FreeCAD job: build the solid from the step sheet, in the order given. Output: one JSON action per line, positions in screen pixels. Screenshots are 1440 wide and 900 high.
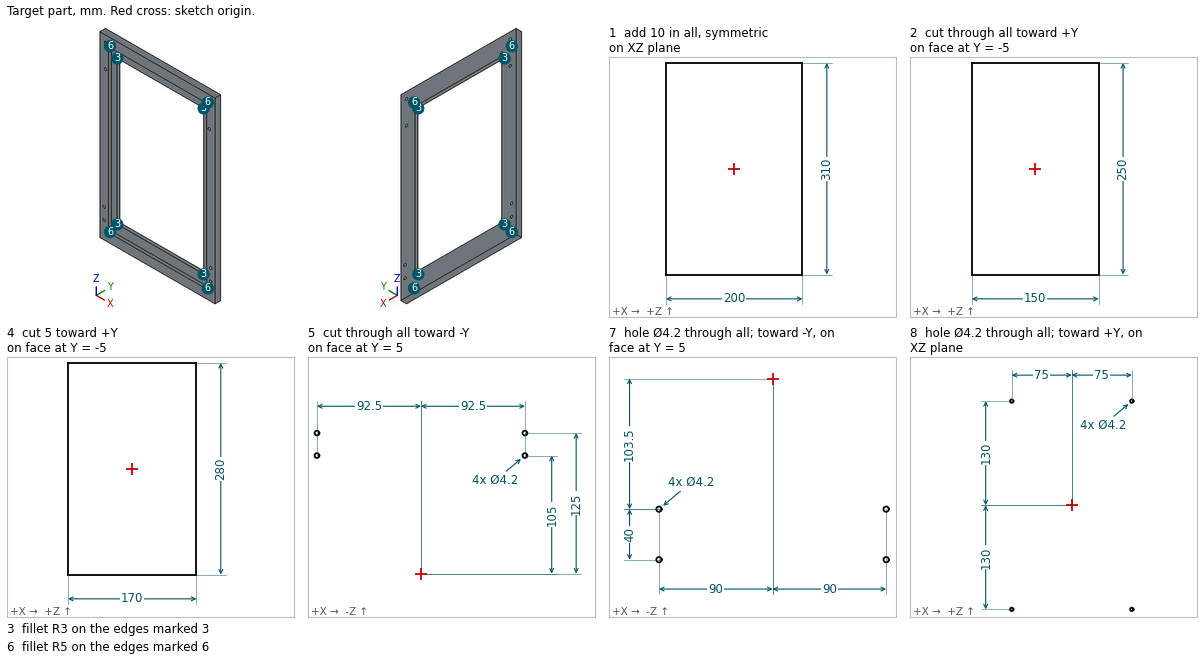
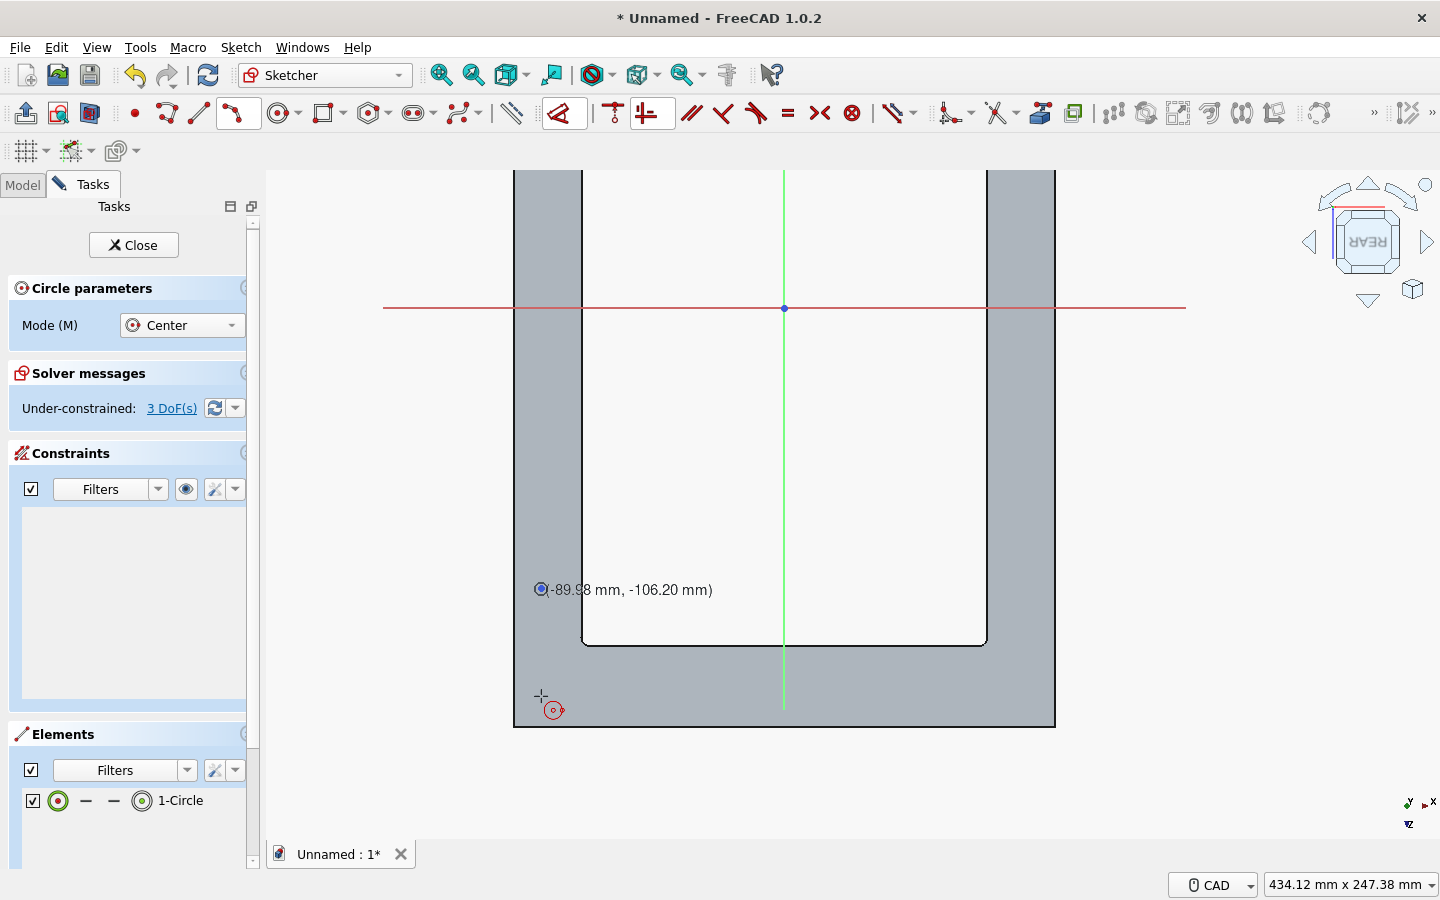
{"action": "left_click", "coordinate": [541, 696]}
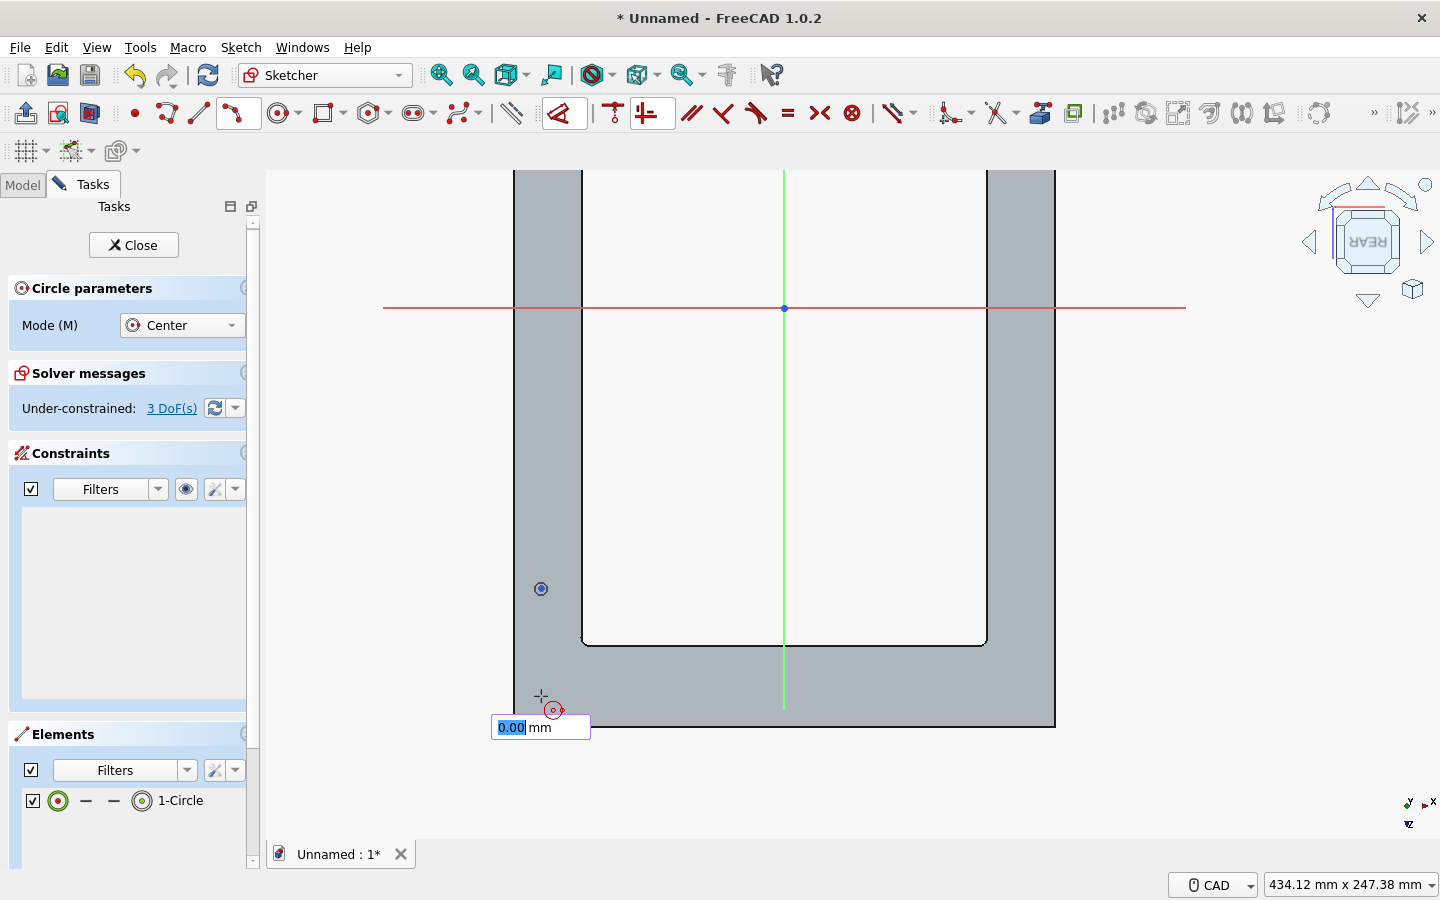
{"action": "scroll", "coordinate": [545, 692], "scroll_direction": "up", "scroll_amount": 6}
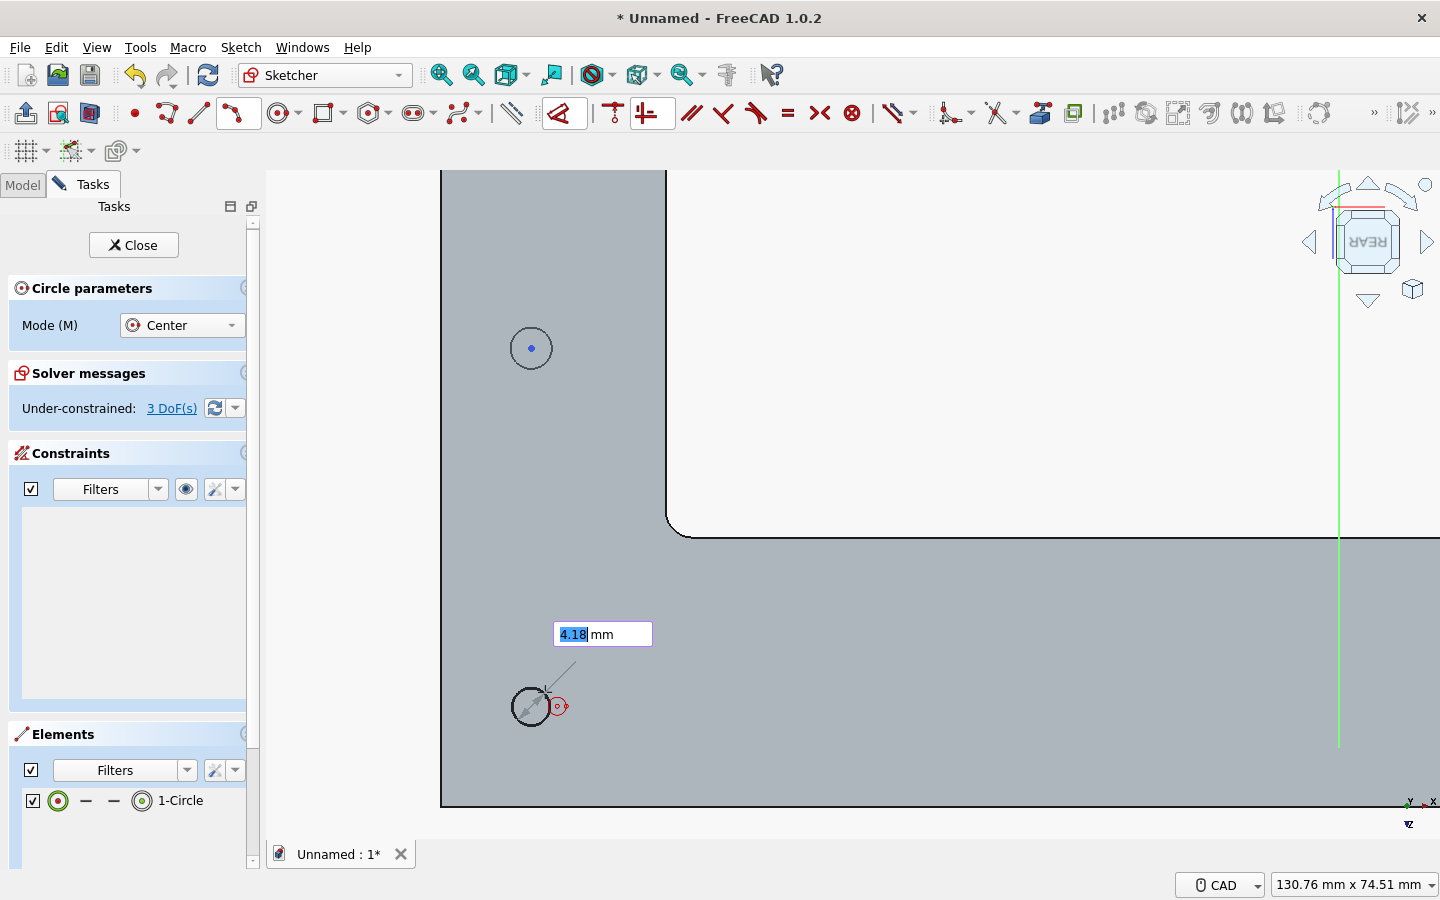
{"action": "left_click", "coordinate": [544, 690]}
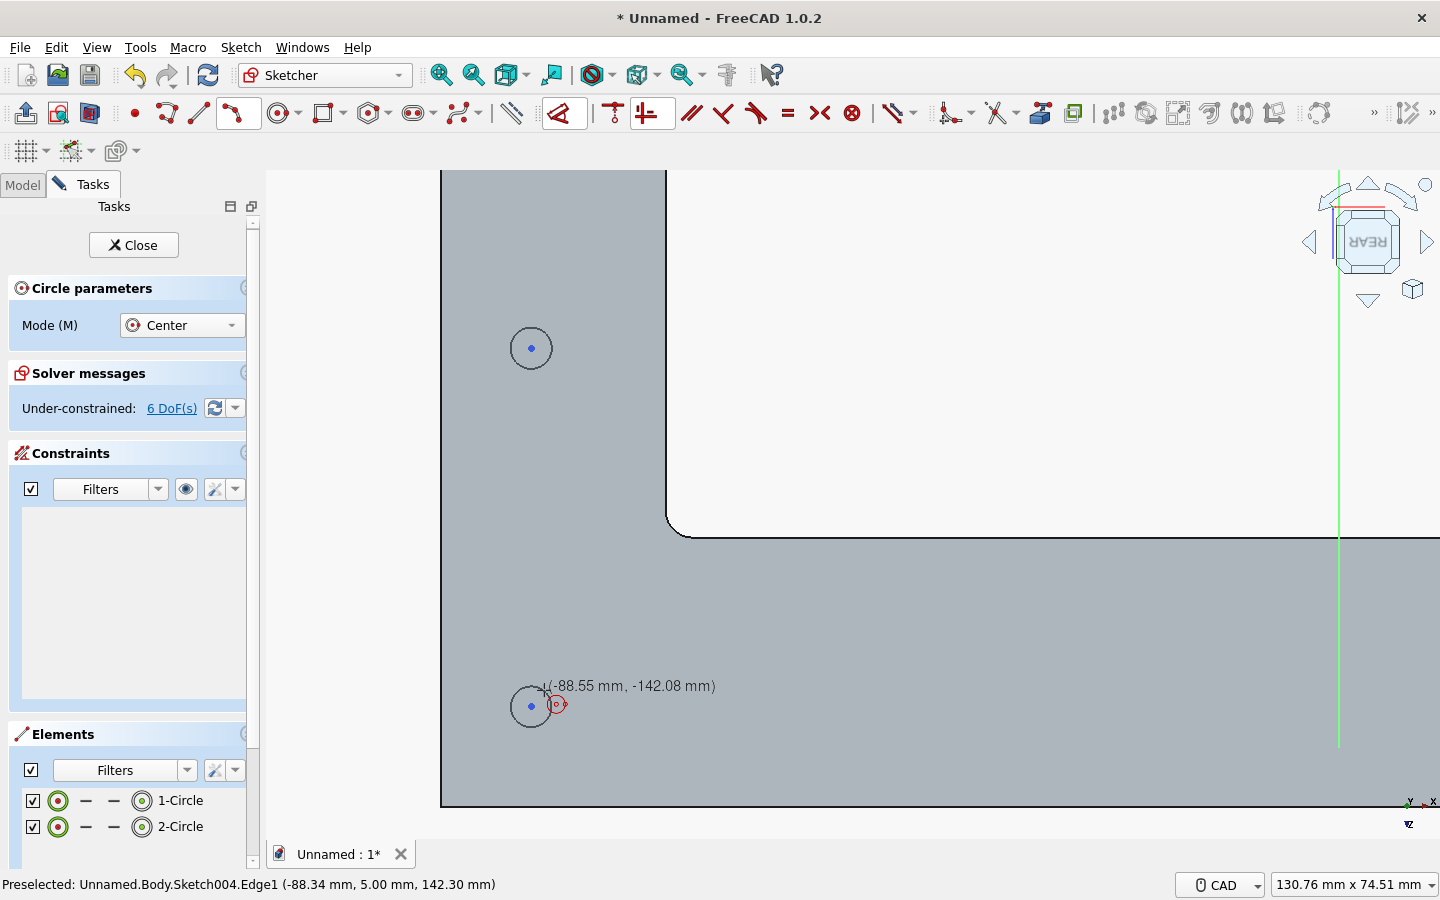
{"action": "scroll", "coordinate": [545, 692], "scroll_direction": "down", "scroll_amount": 6}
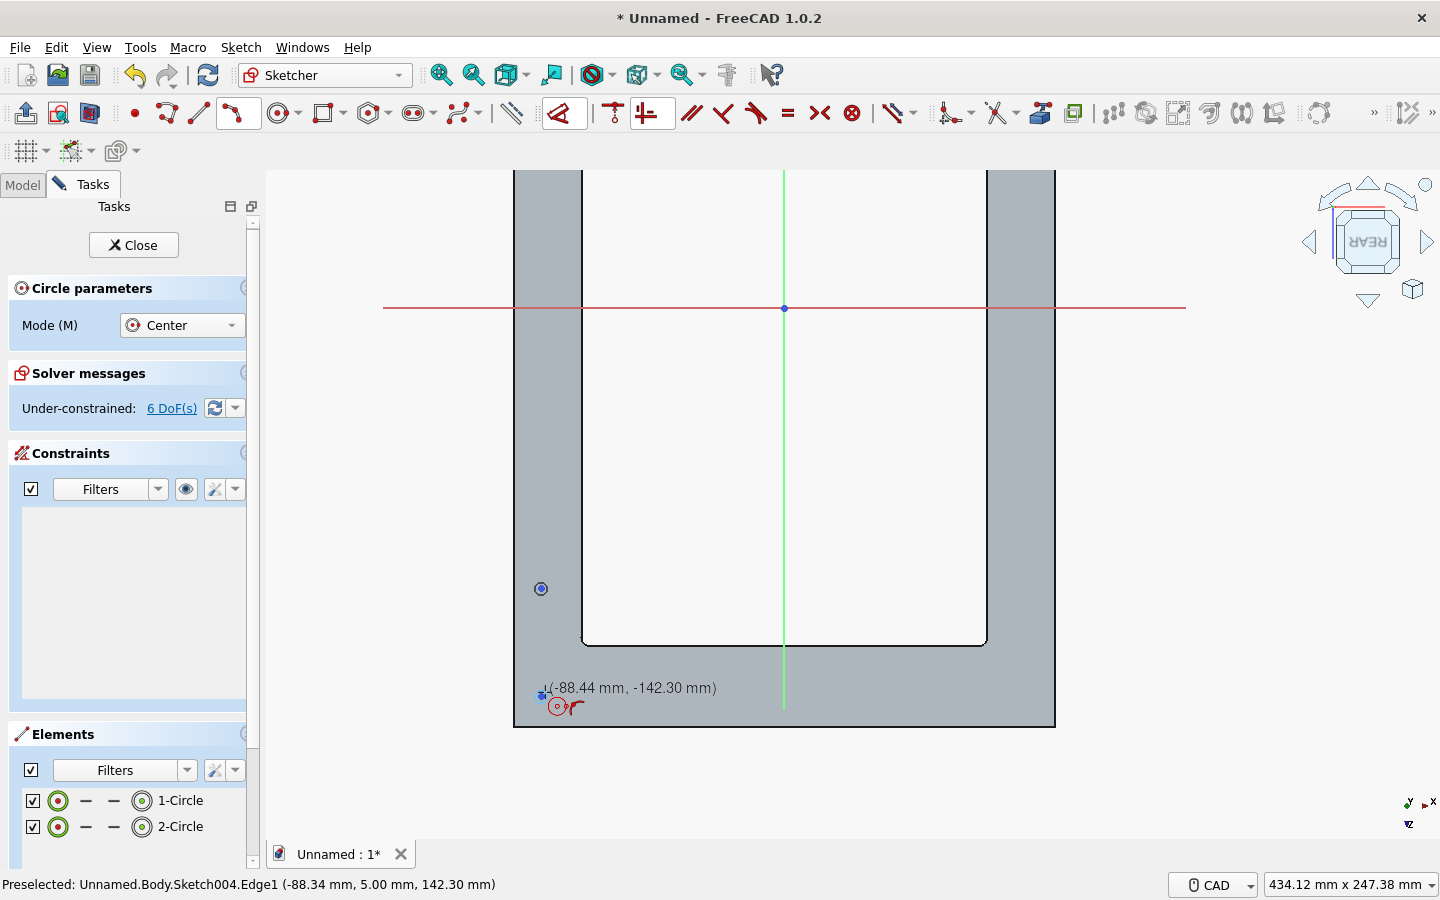
{"action": "scroll", "coordinate": [1028, 588], "scroll_direction": "up", "scroll_amount": 7}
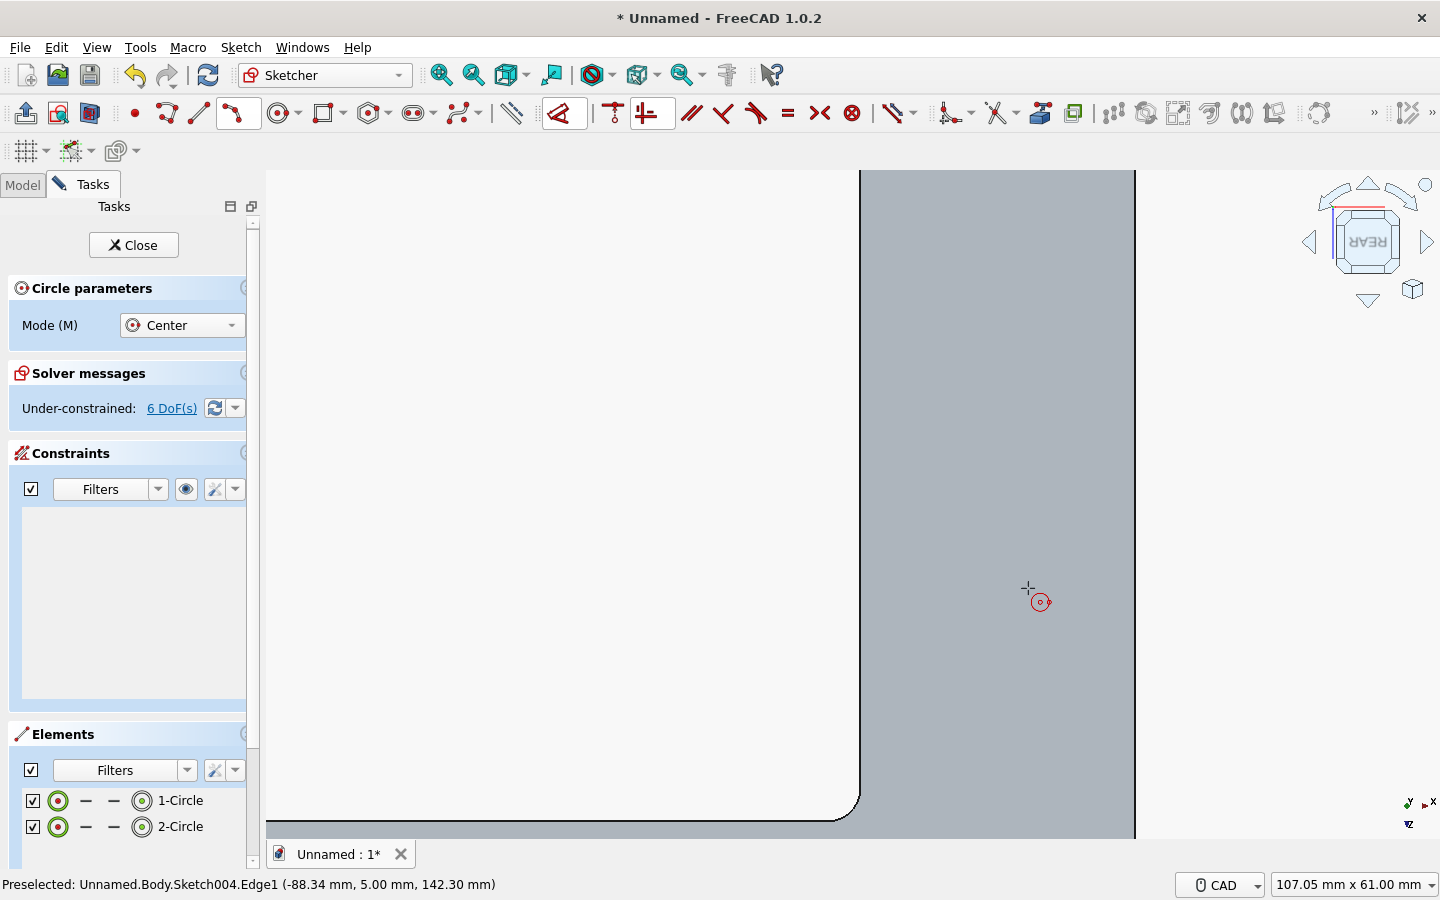
{"action": "scroll", "coordinate": [1029, 588], "scroll_direction": "down", "scroll_amount": 7}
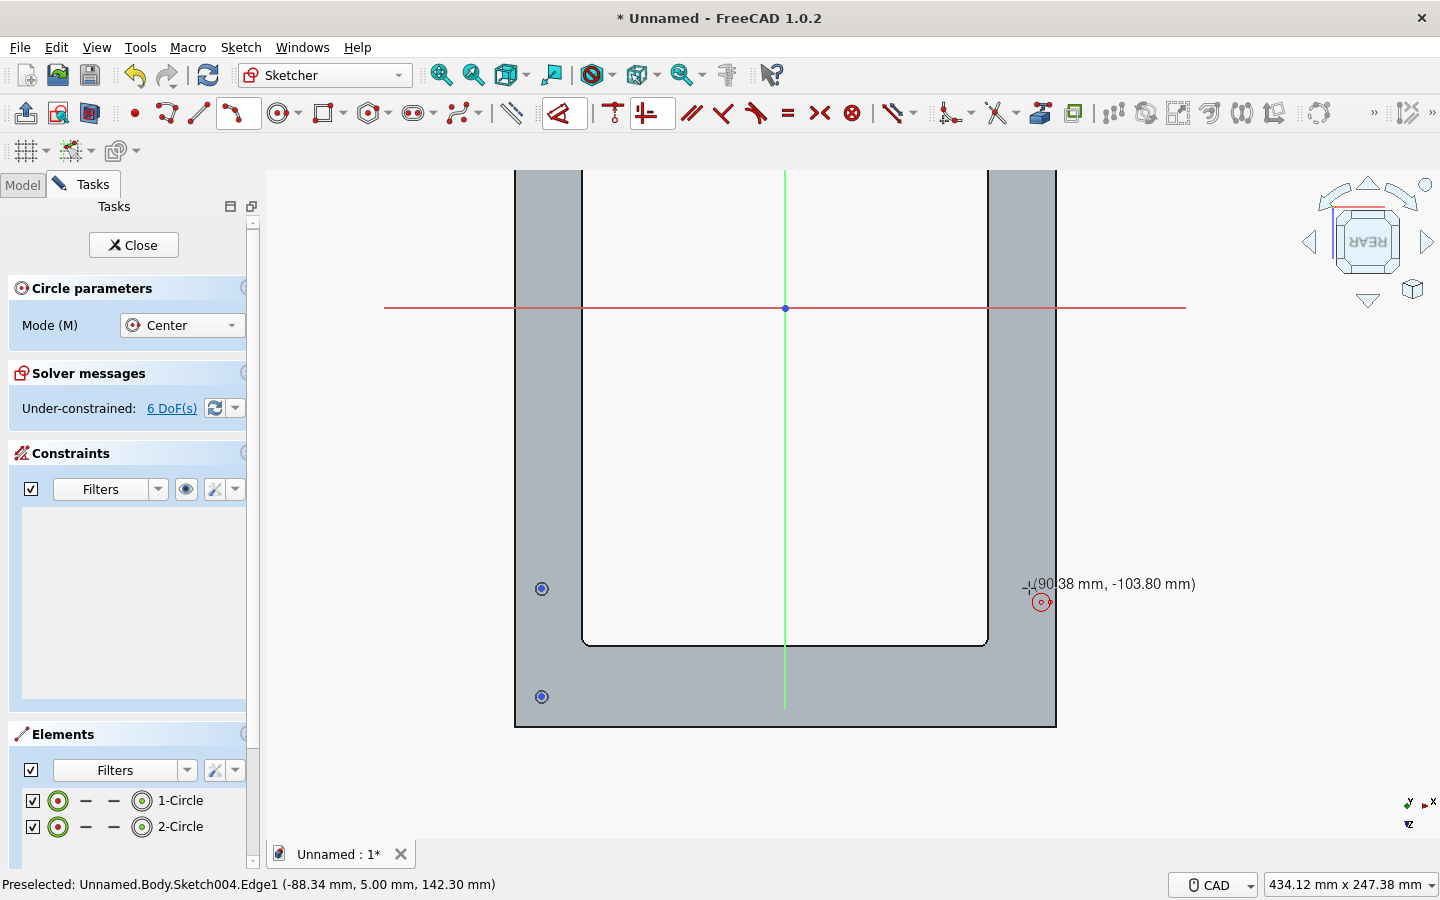
{"action": "left_click", "coordinate": [1028, 588]}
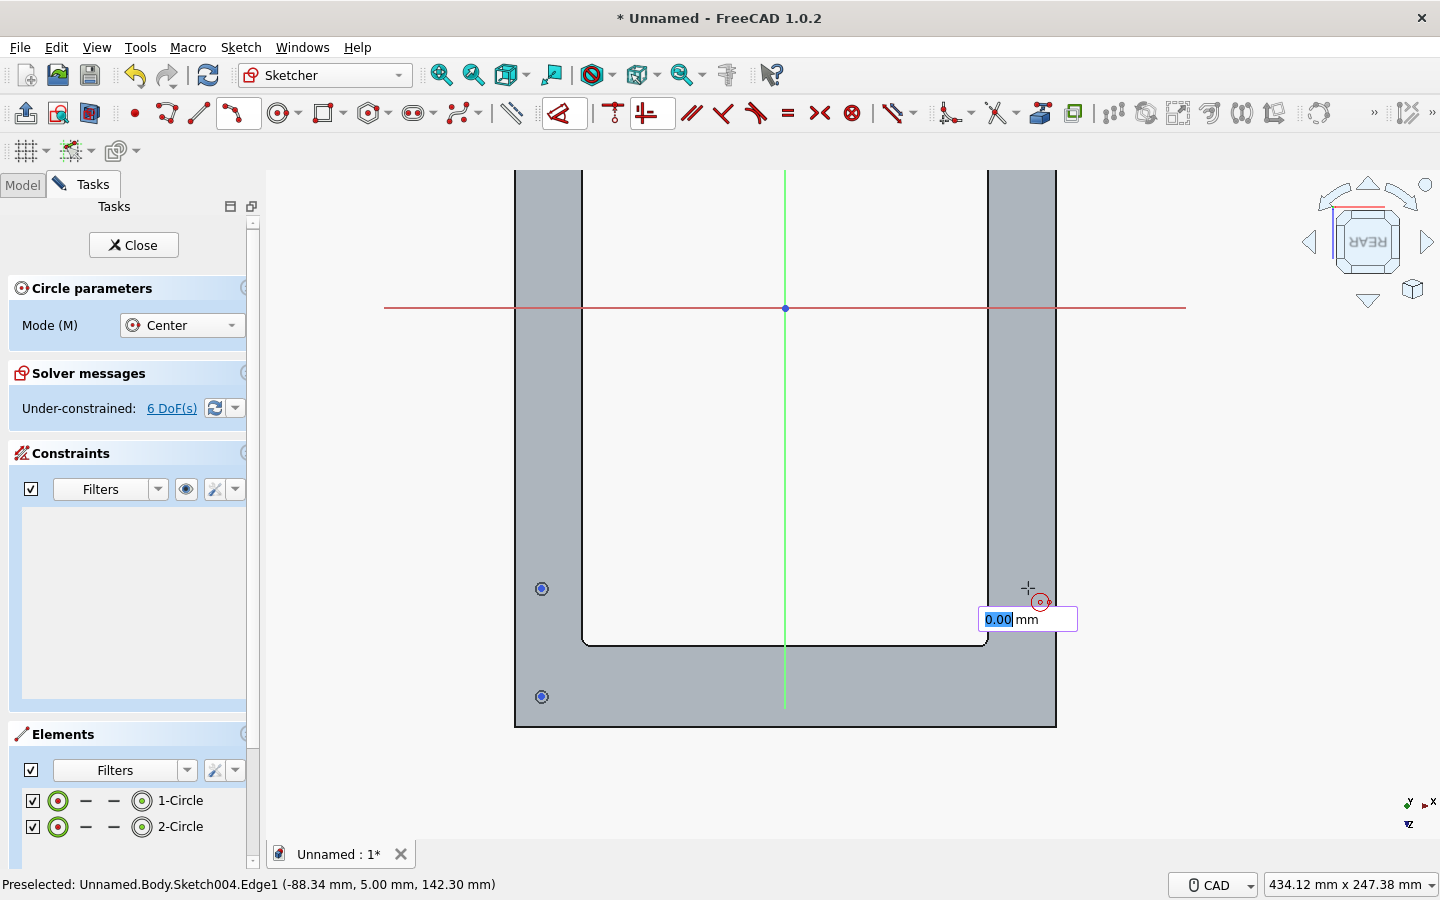
{"action": "scroll", "coordinate": [1032, 584], "scroll_direction": "up", "scroll_amount": 6}